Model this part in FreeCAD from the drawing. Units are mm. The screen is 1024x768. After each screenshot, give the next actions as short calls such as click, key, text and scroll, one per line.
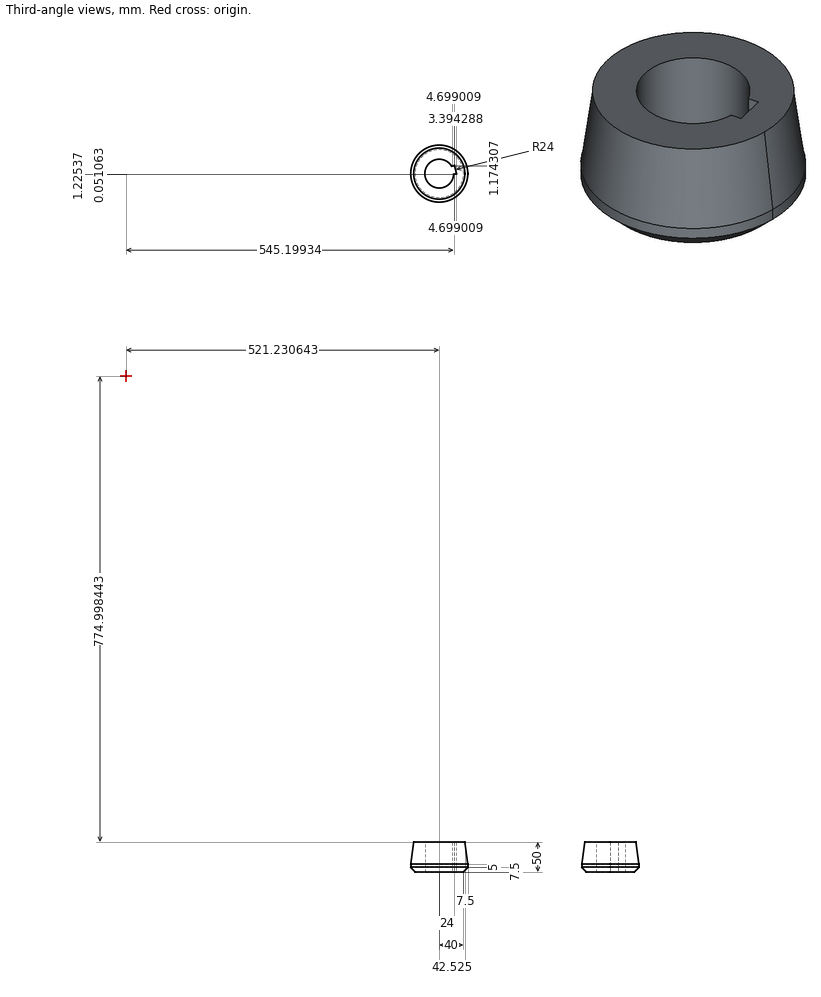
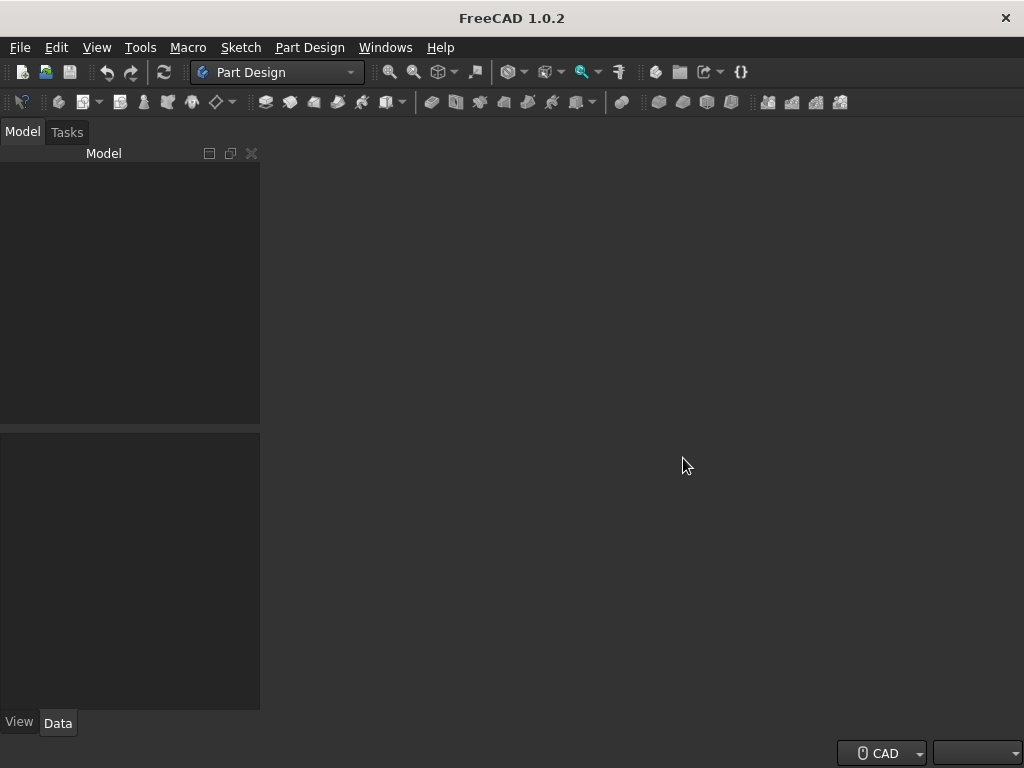
click(22, 72)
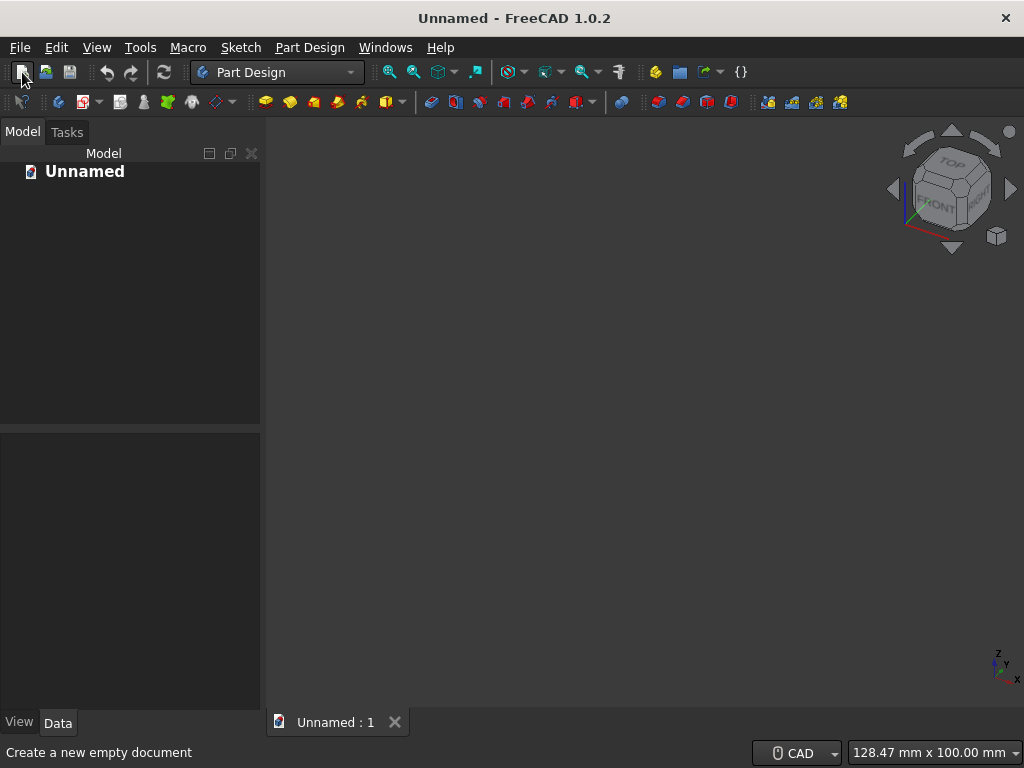
click(60, 102)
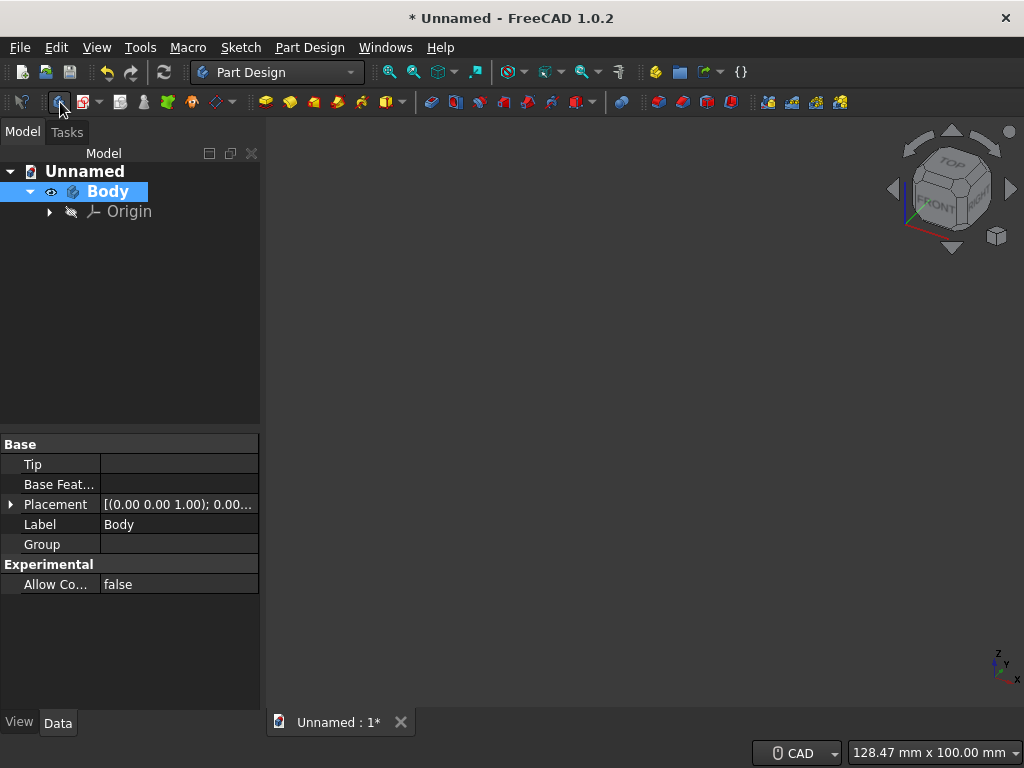
click(50, 212)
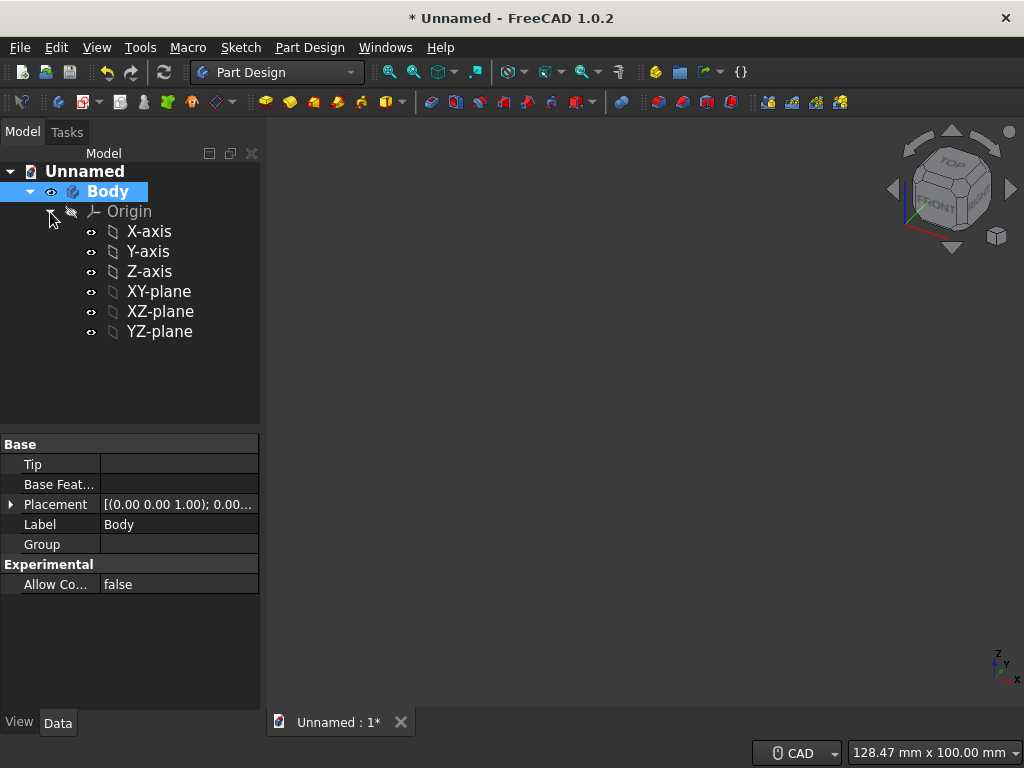
click(136, 312)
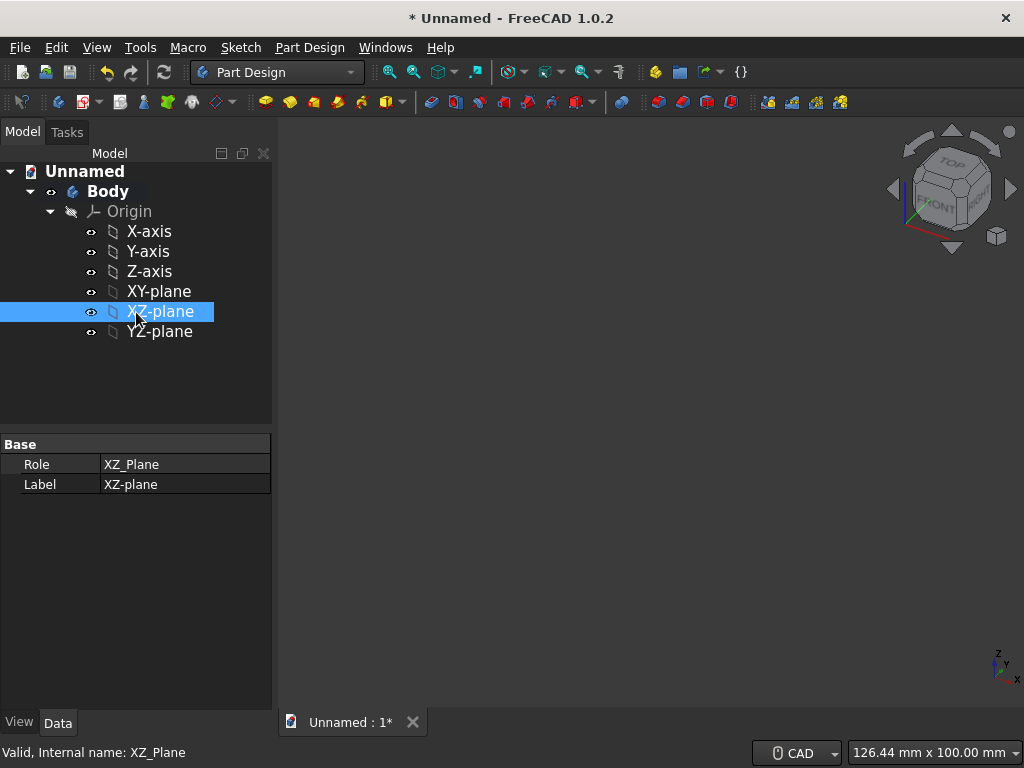
click(216, 102)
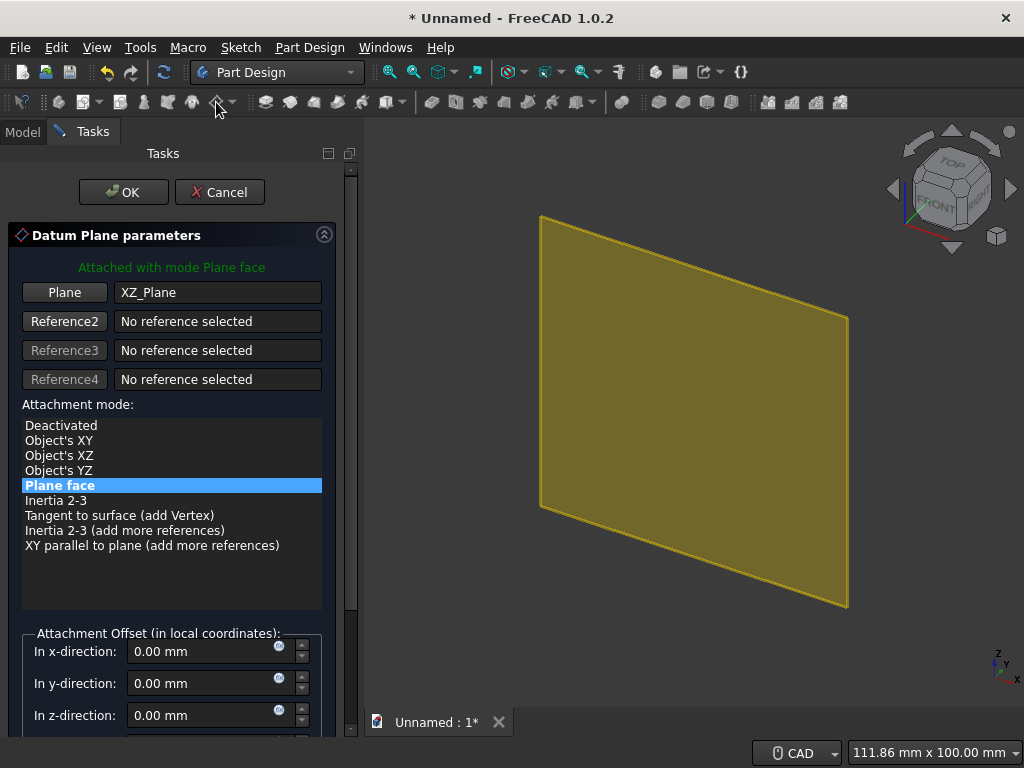
triple_click(210, 715)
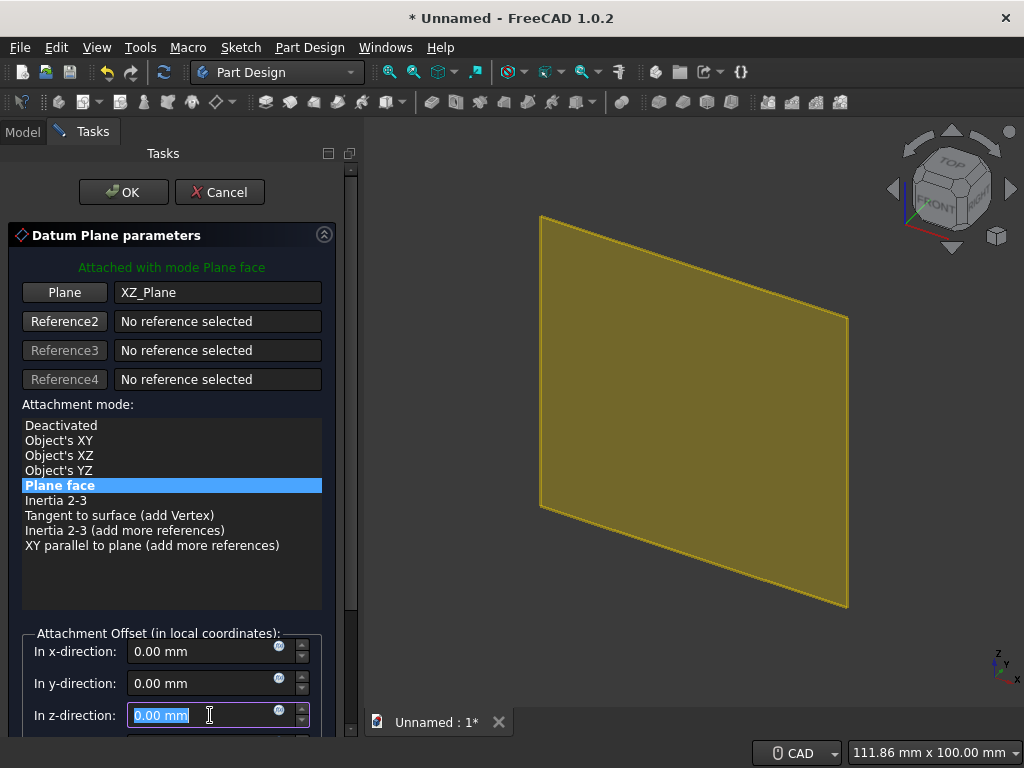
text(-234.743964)
key(Tab)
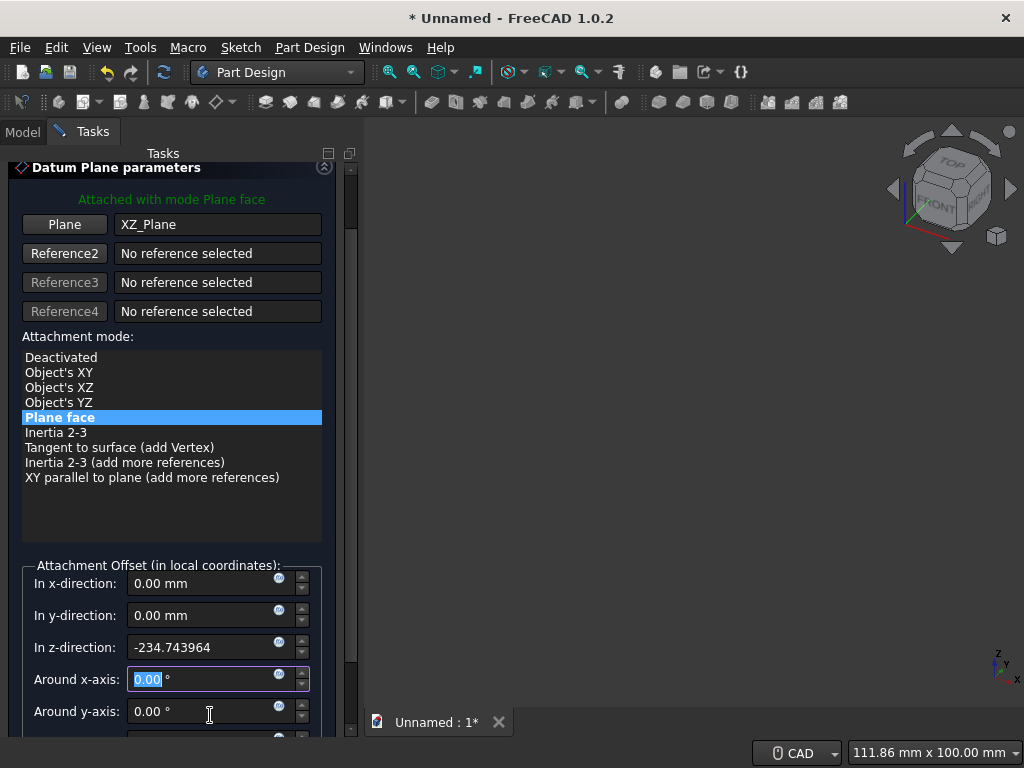
scroll(351, 450, up, 2)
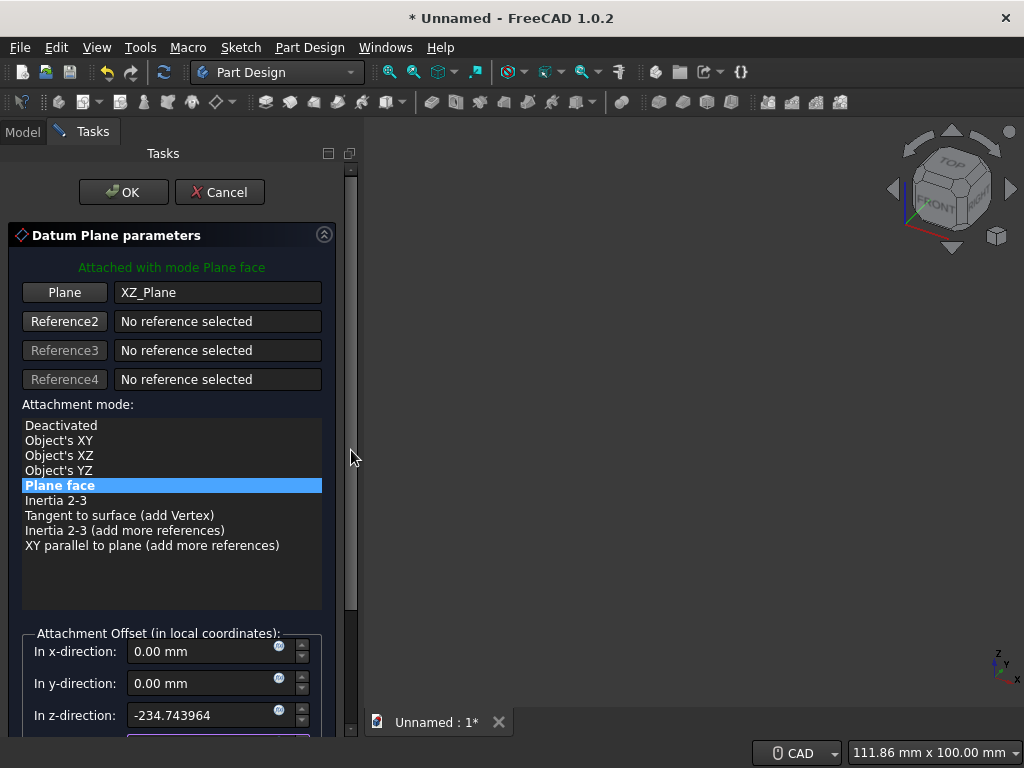
click(124, 192)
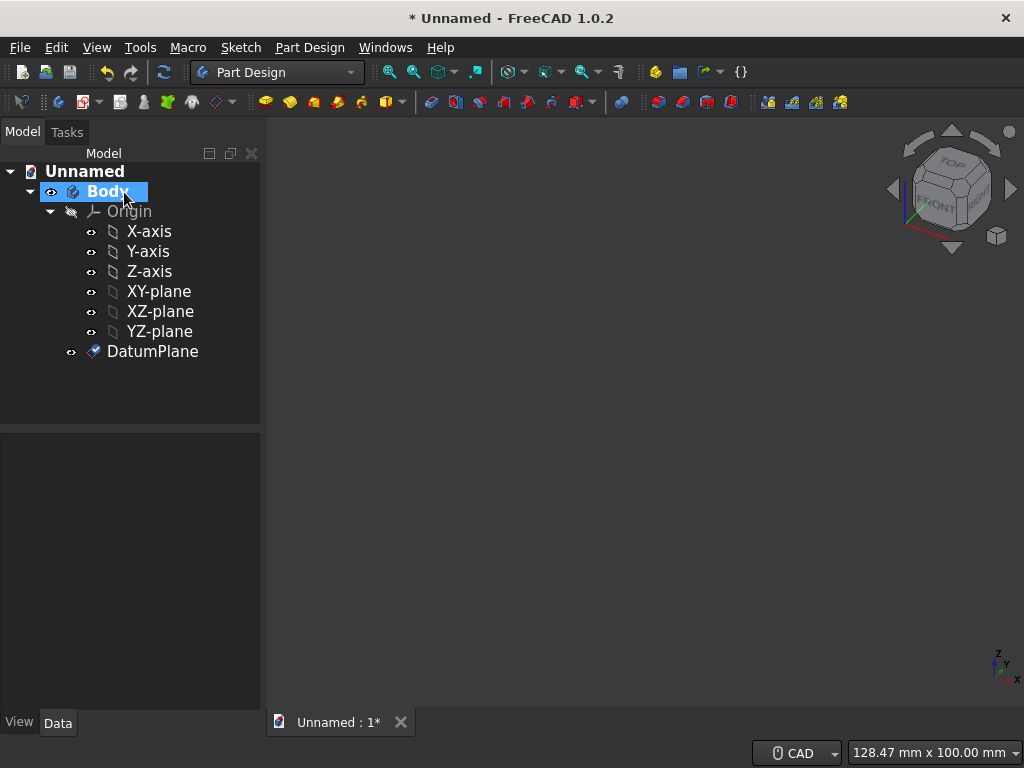
click(116, 352)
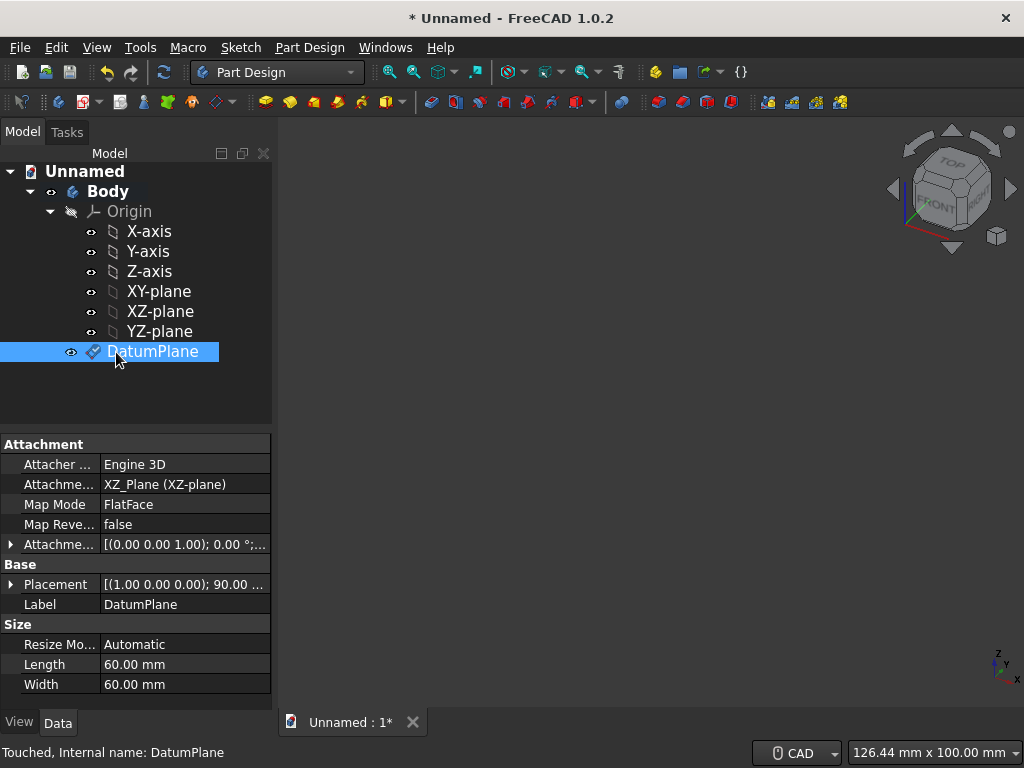
click(84, 102)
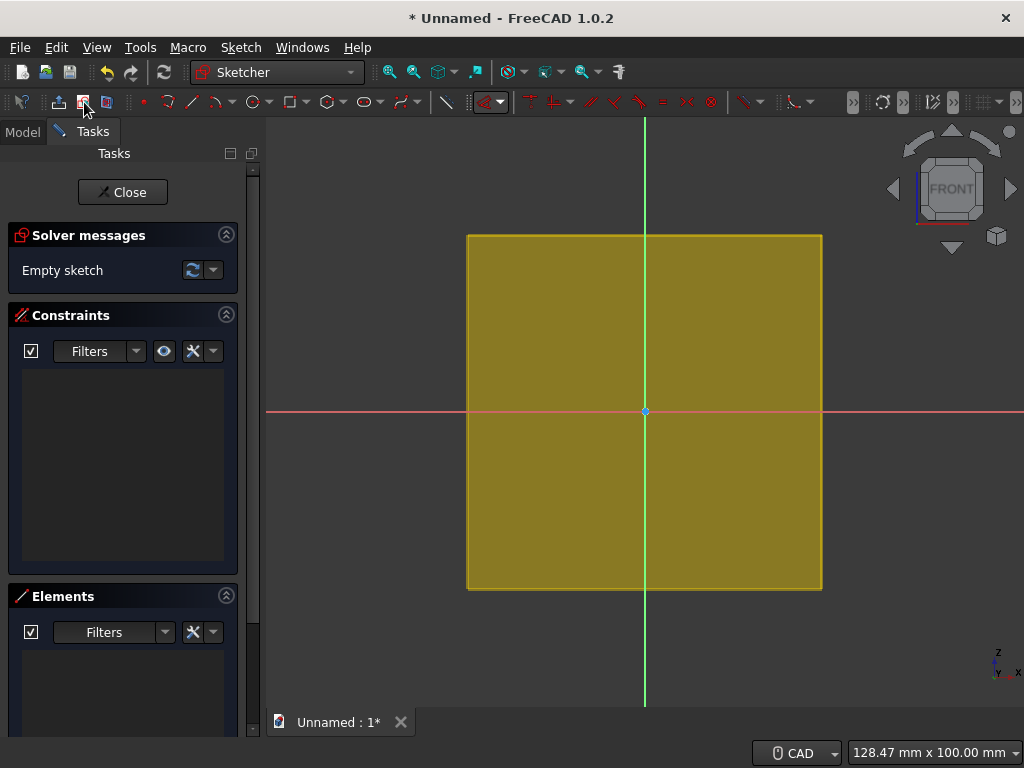
scroll(576, 412, down, 5)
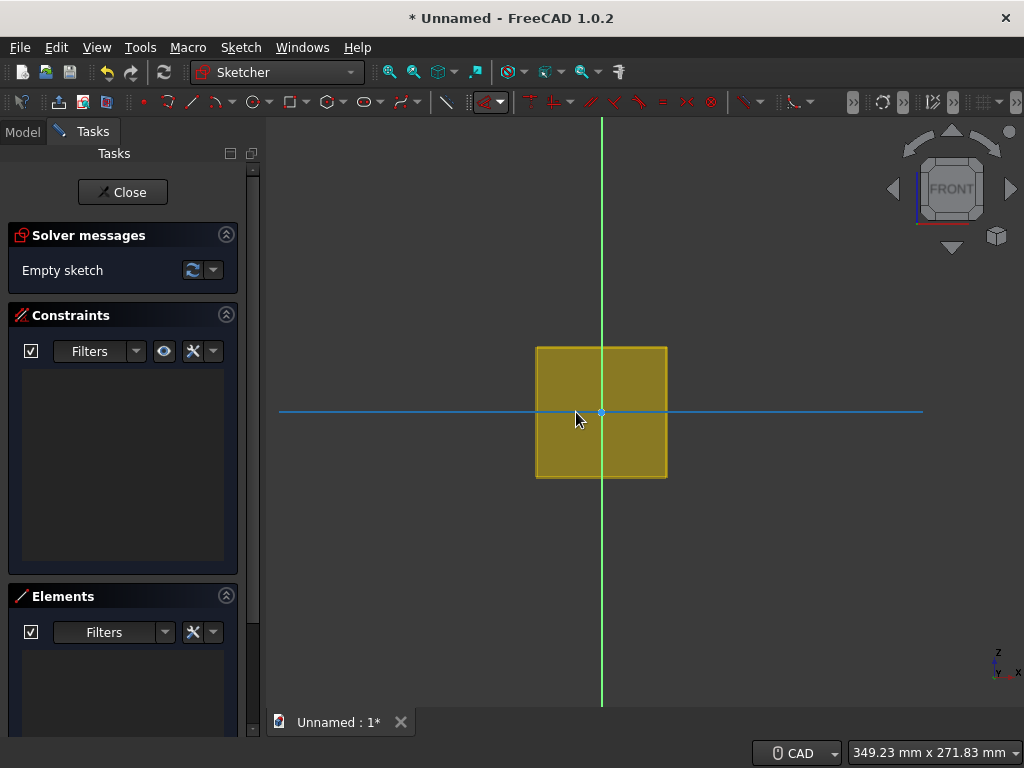
scroll(576, 412, down, 5)